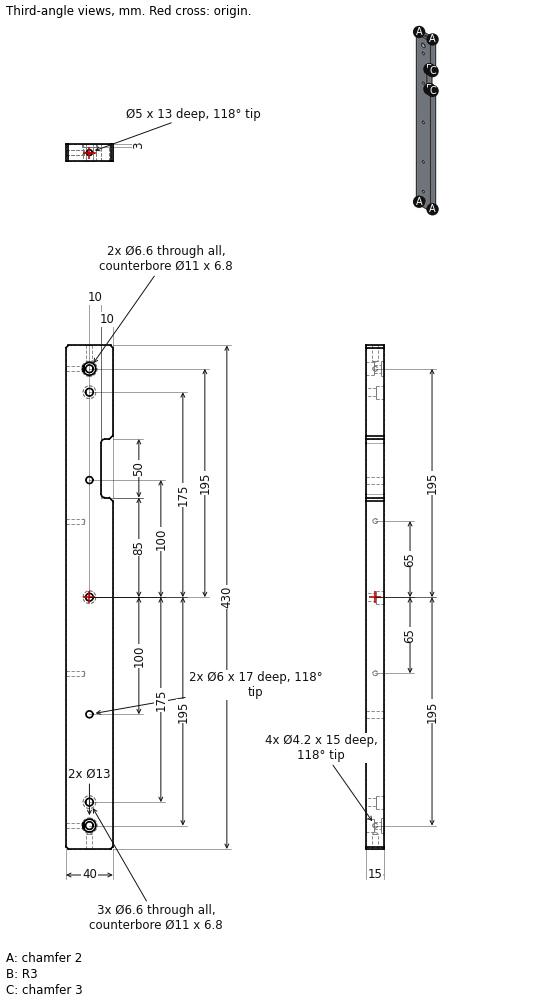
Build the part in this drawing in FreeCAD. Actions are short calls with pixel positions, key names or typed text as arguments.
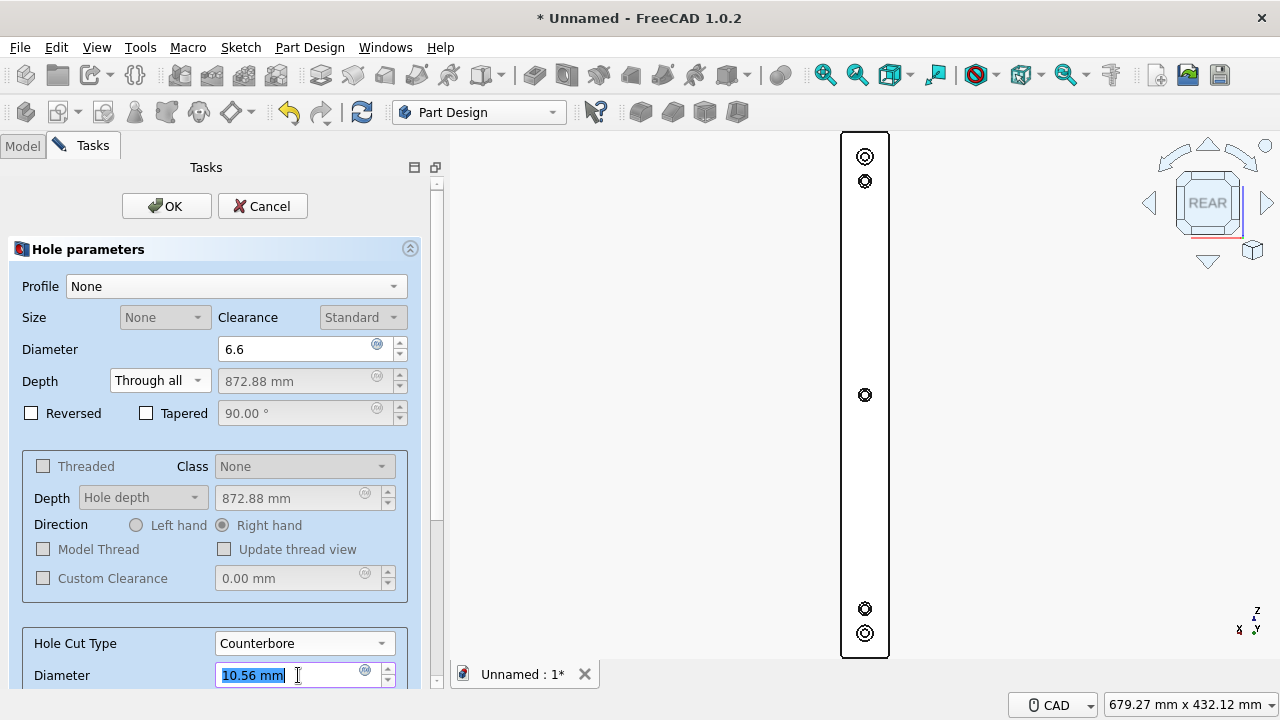
text(11)
key(Tab)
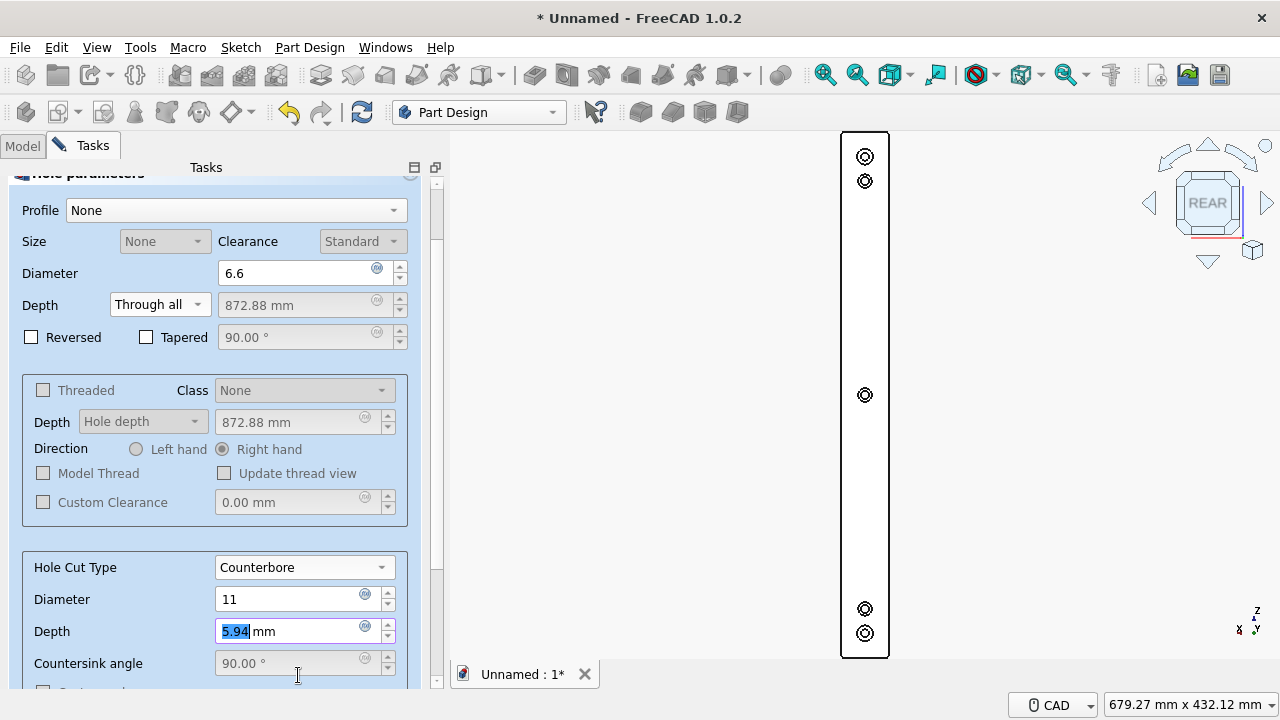
text(6.8)
key(Tab)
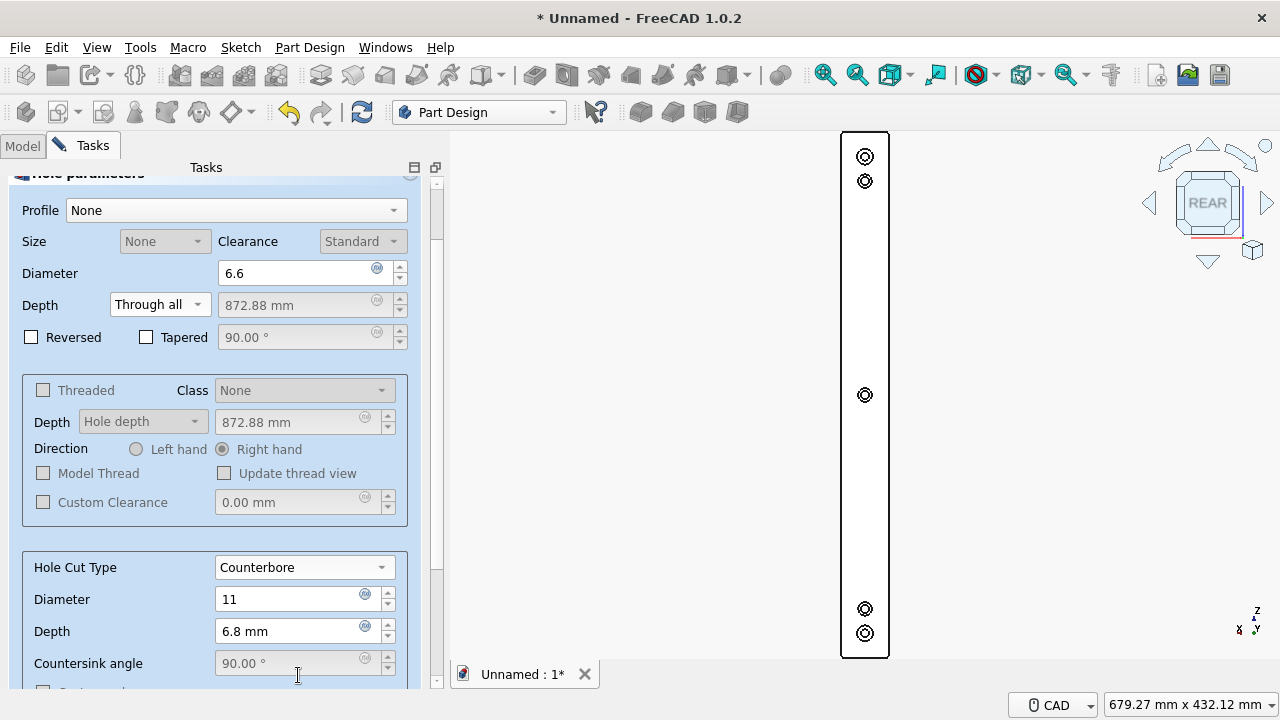
scroll(437, 432, up, 3)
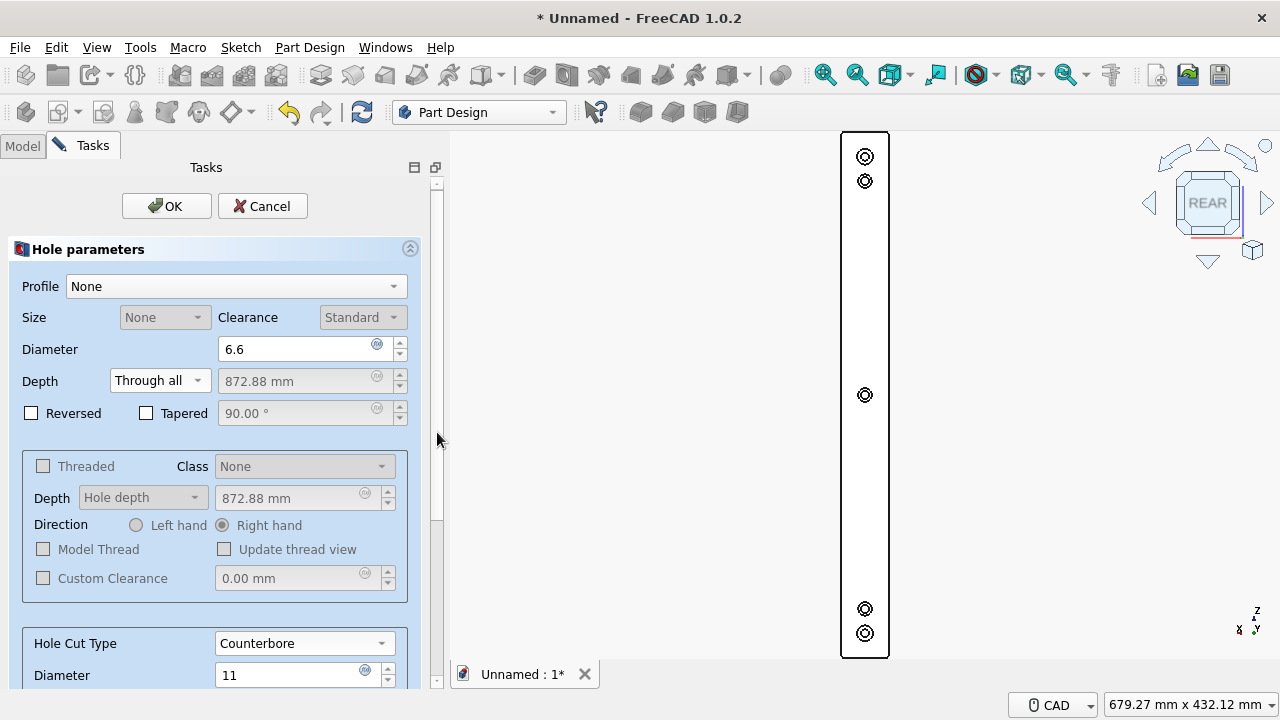
click(167, 206)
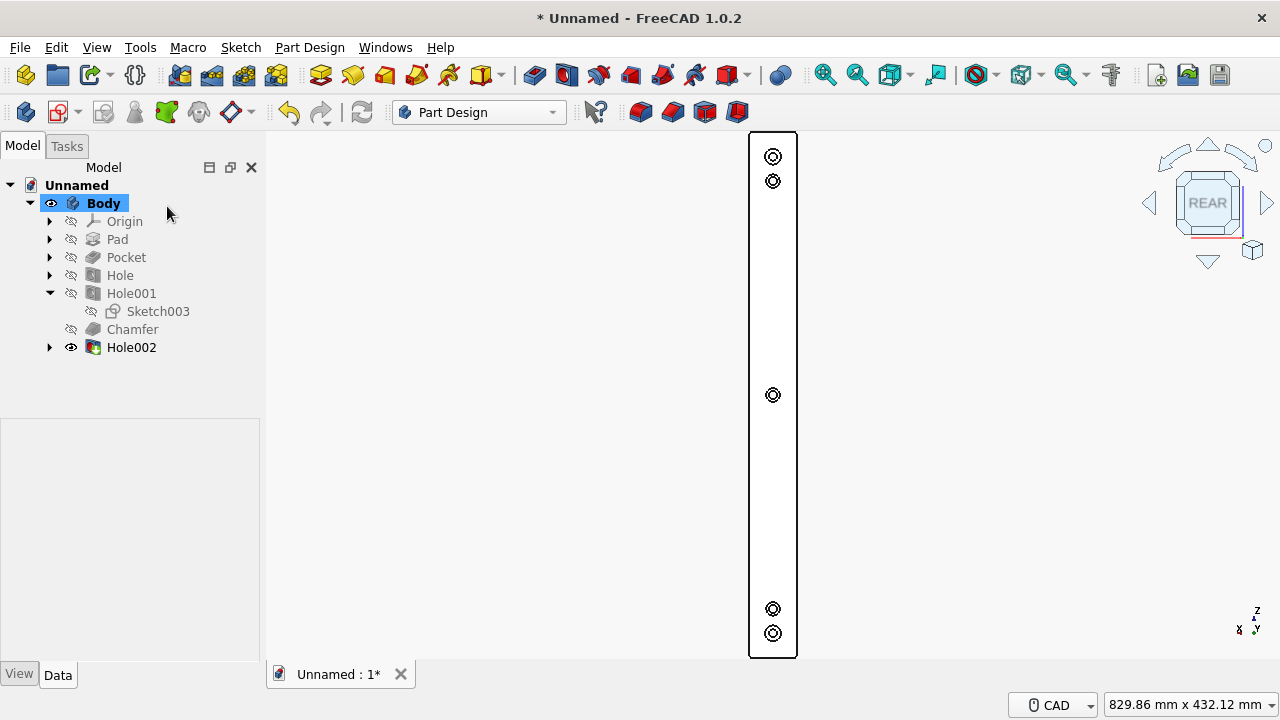
key(0)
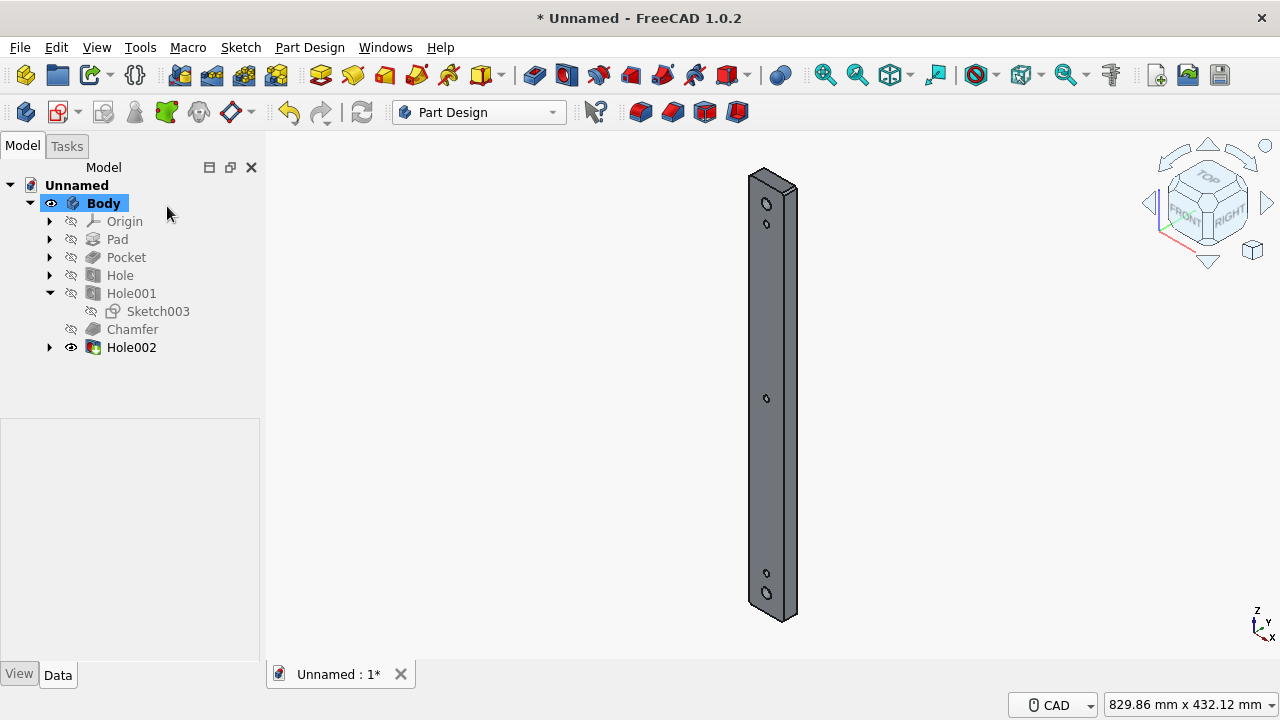
key(2)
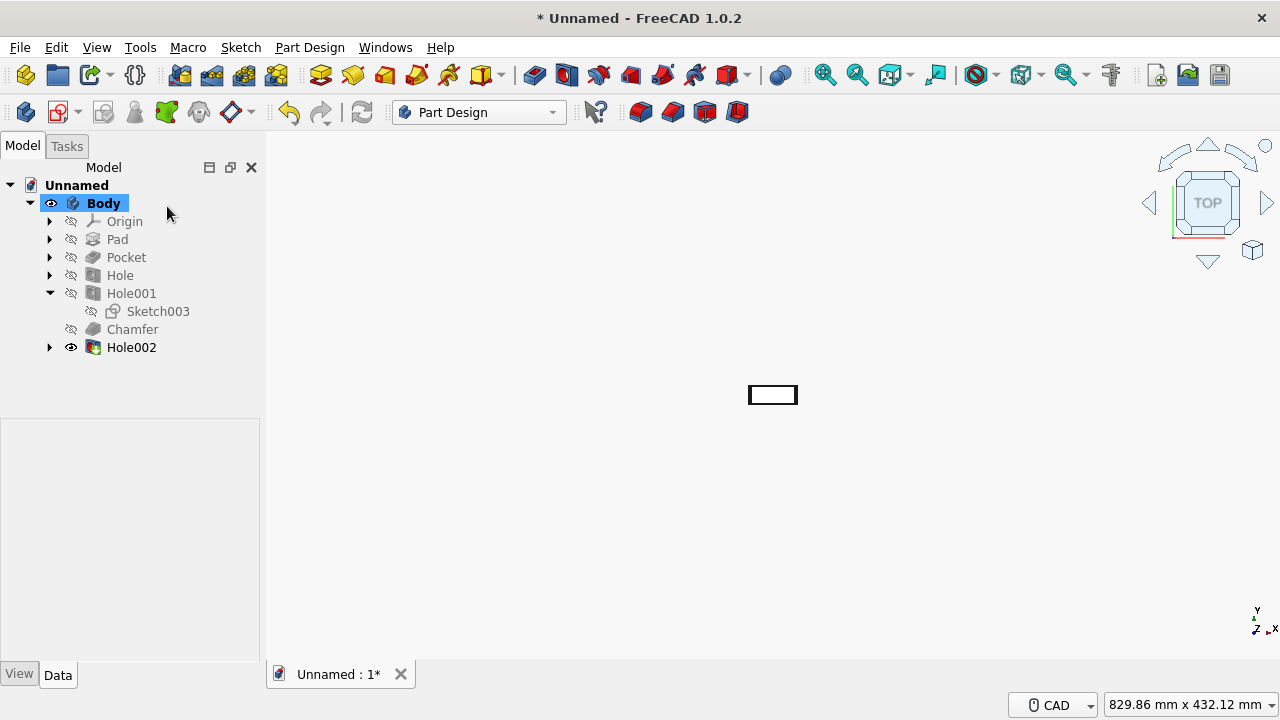
click(826, 76)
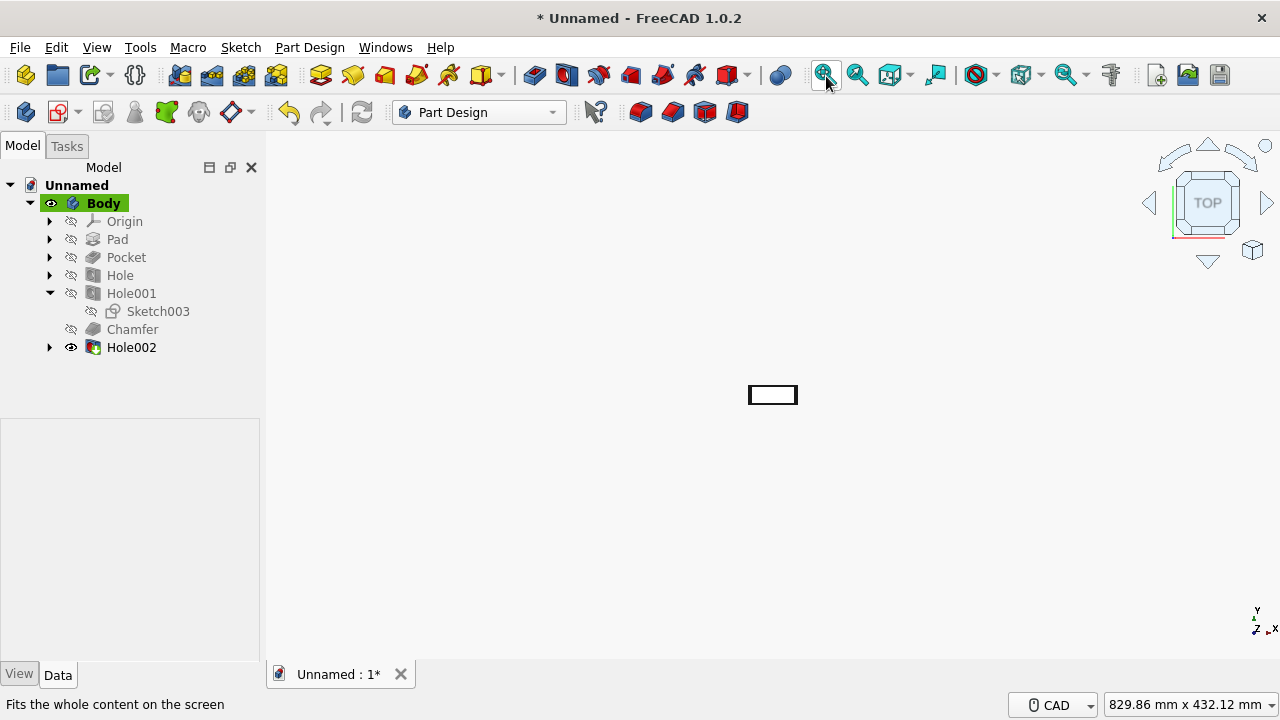
click(786, 394)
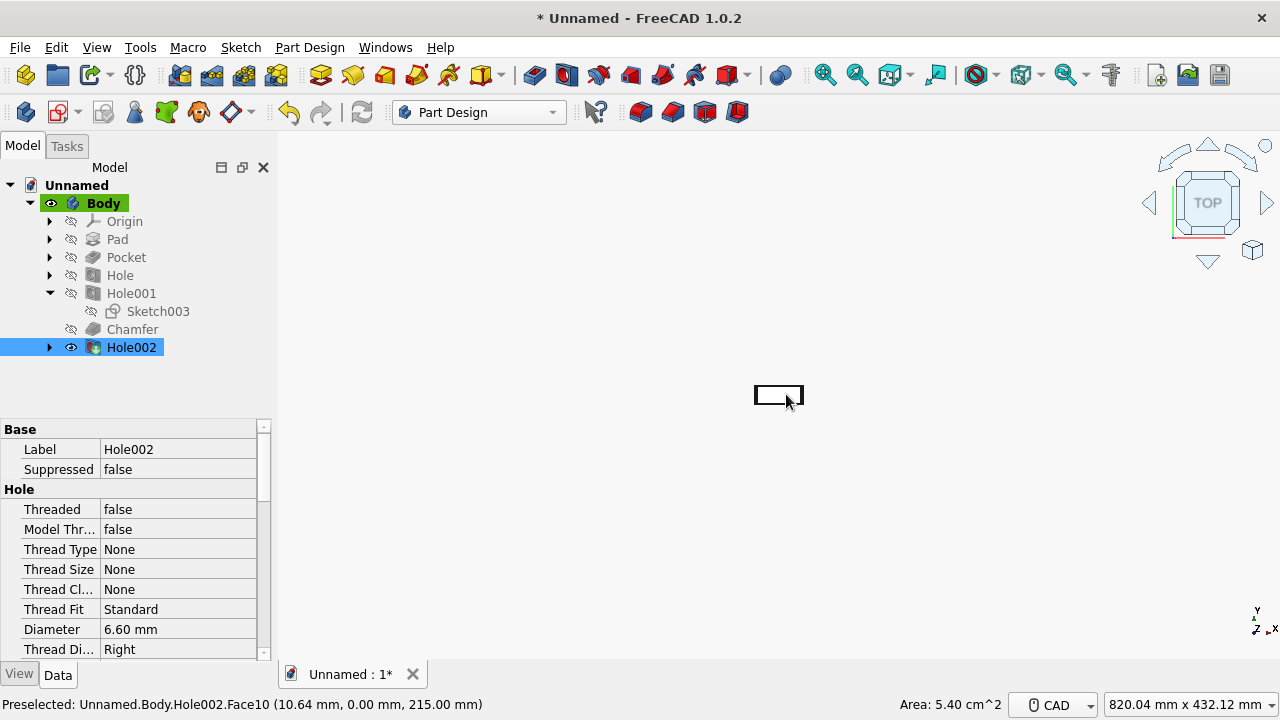
click(58, 112)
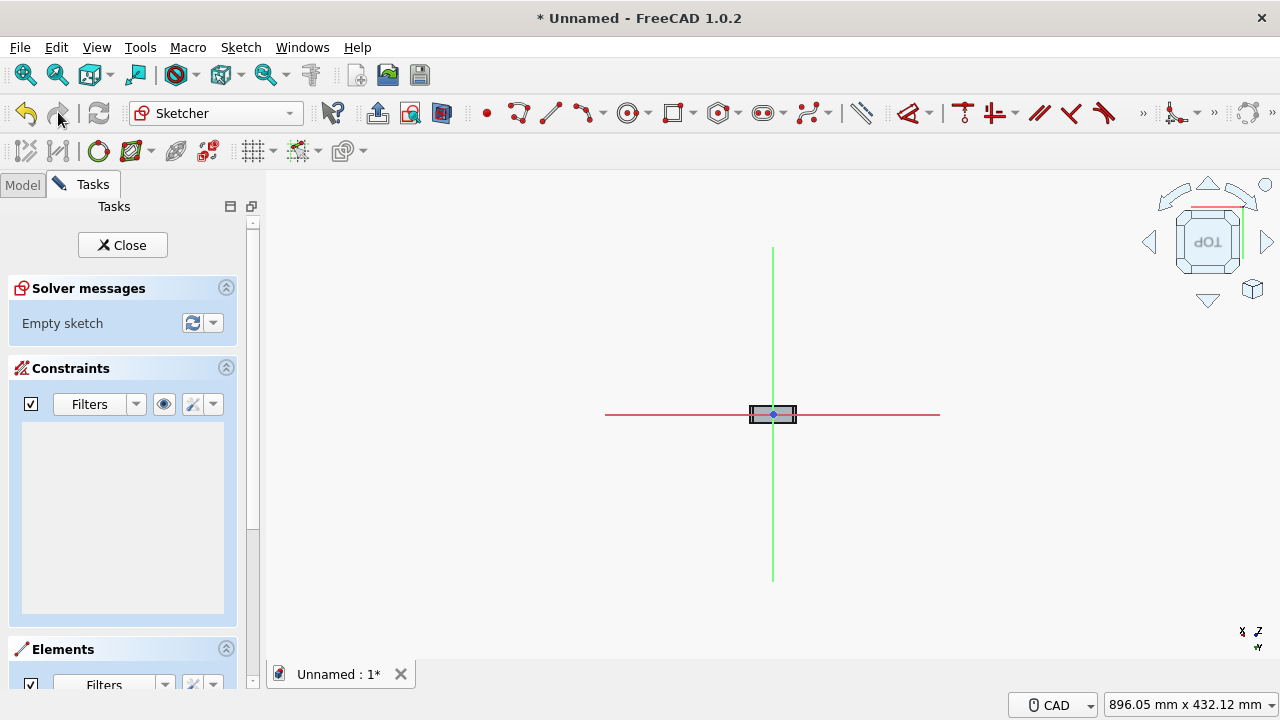
scroll(777, 415, up, 15)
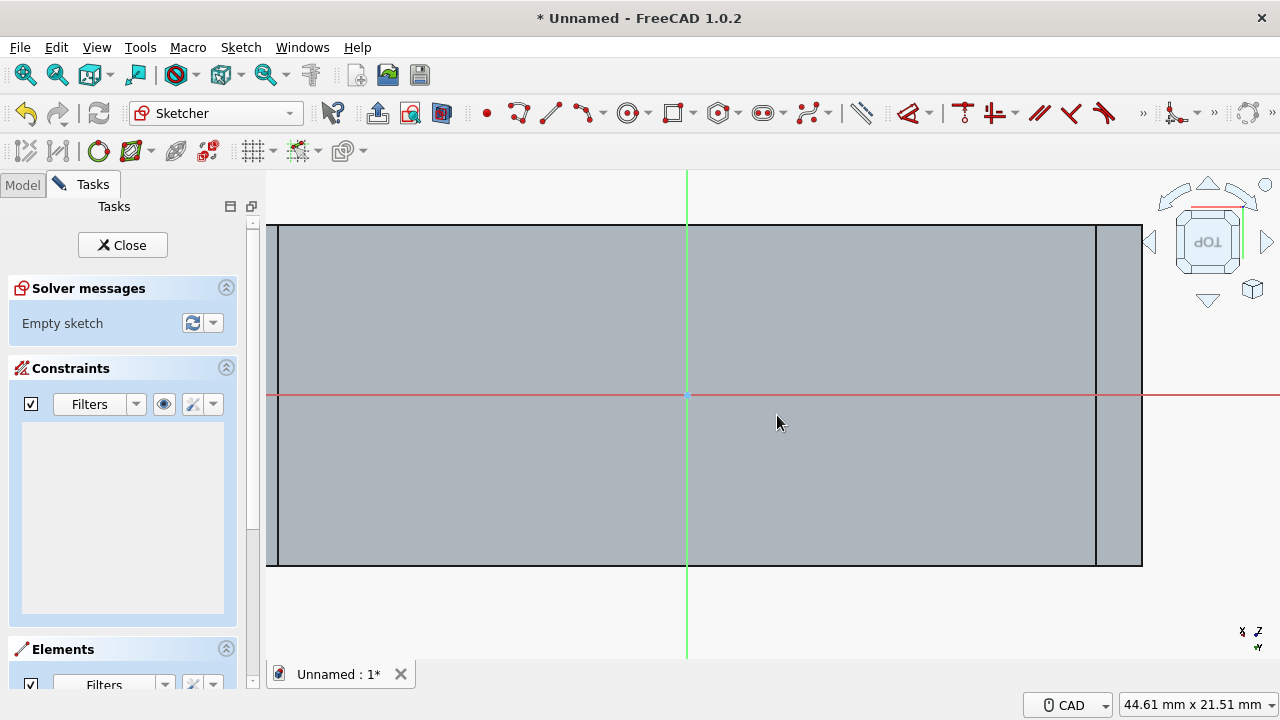
scroll(677, 384, up, 5)